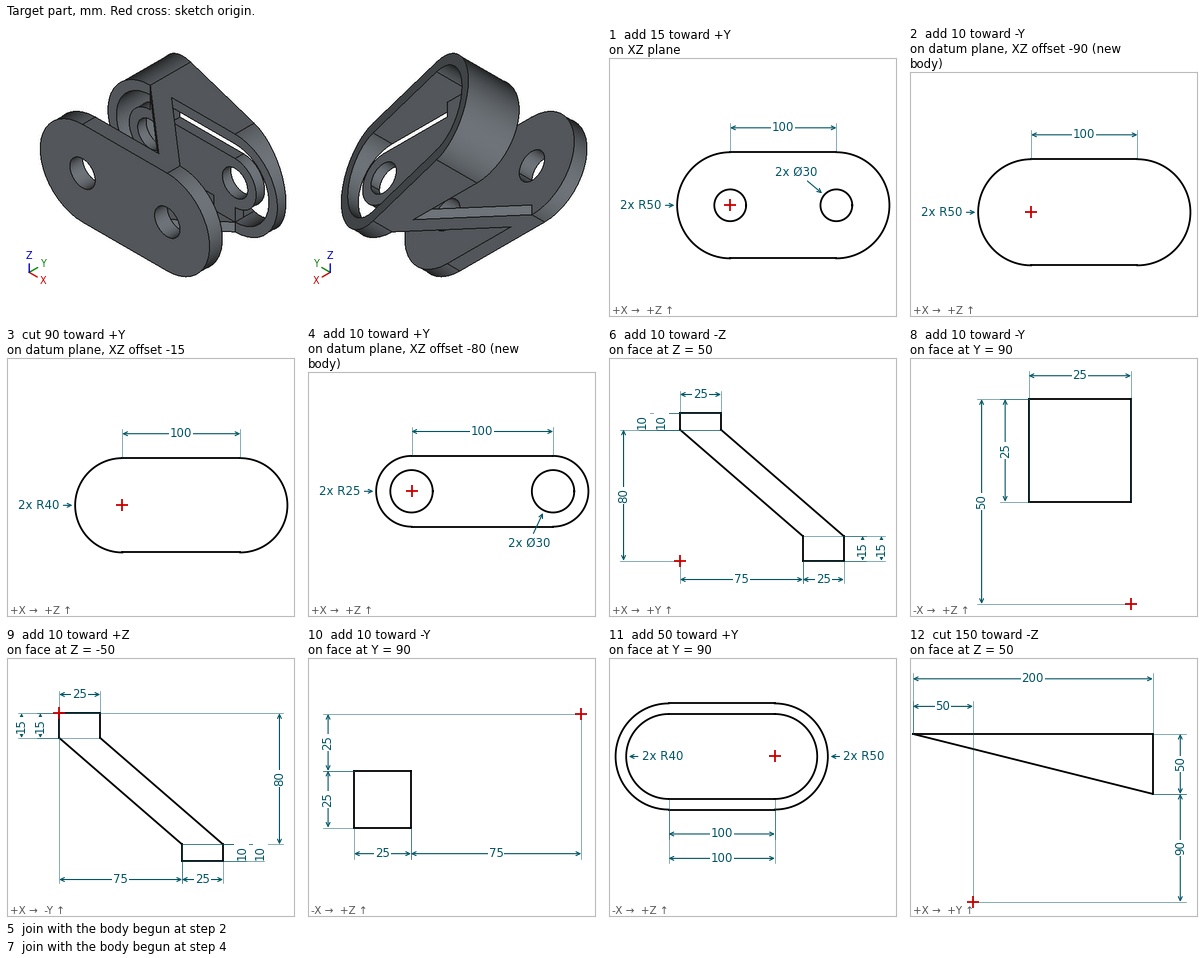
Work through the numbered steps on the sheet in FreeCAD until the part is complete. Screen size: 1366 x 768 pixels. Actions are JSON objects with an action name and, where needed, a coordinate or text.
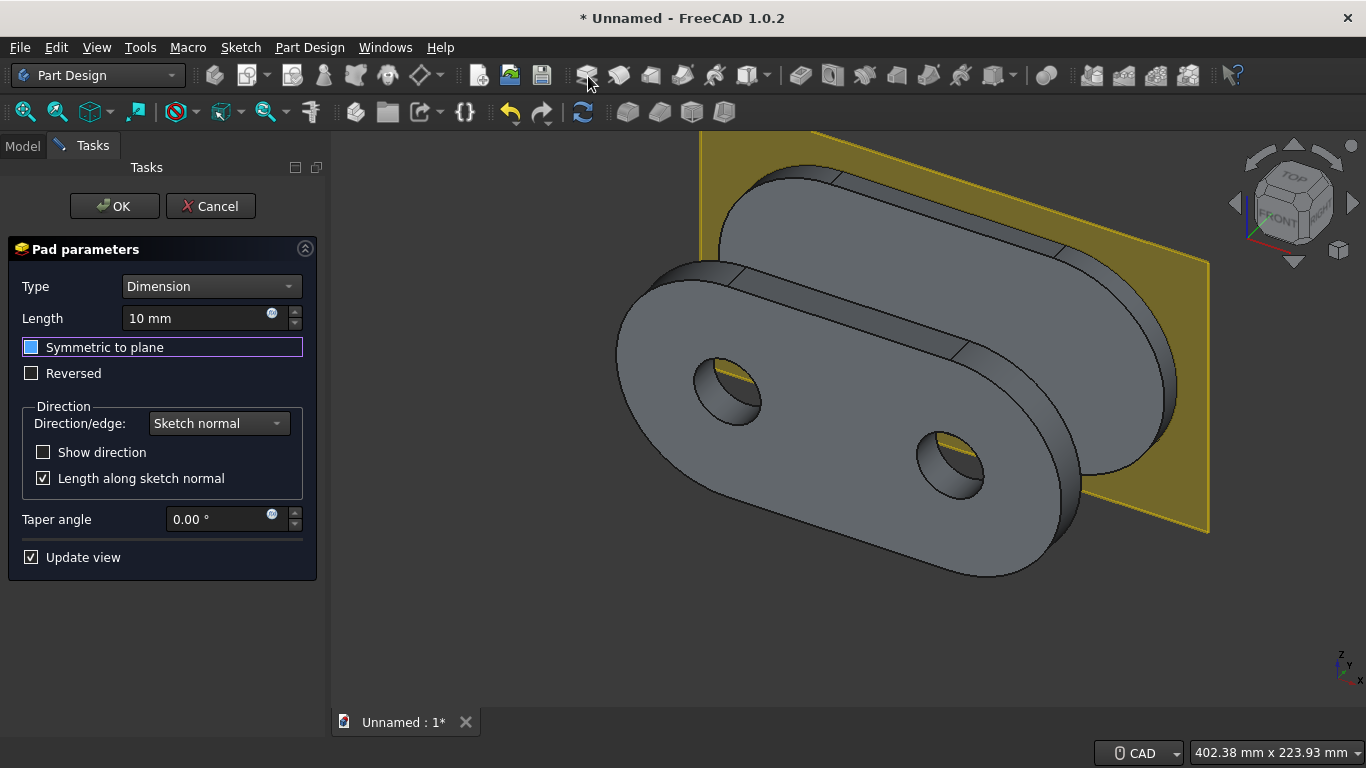
{"action": "left_click", "coordinate": [115, 206]}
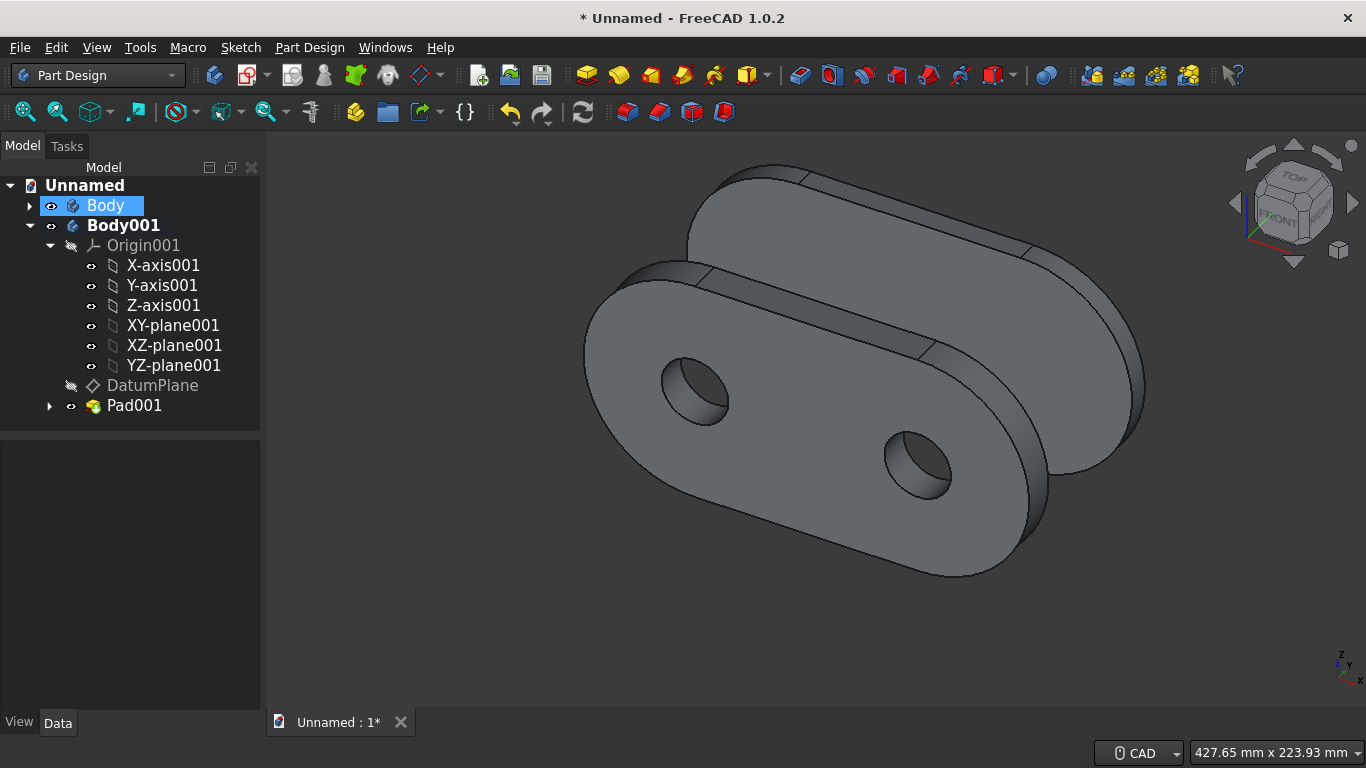
{"action": "left_click", "coordinate": [136, 346]}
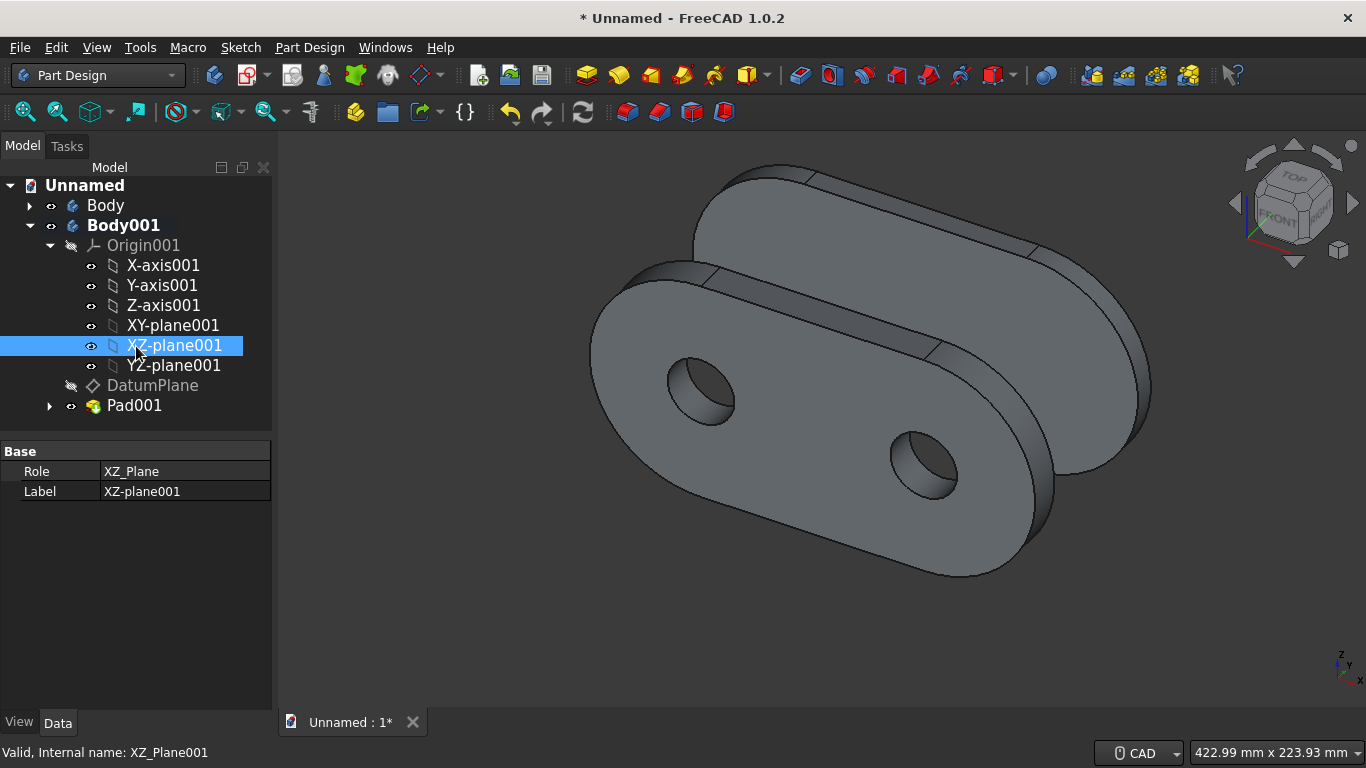
{"action": "left_click", "coordinate": [420, 76]}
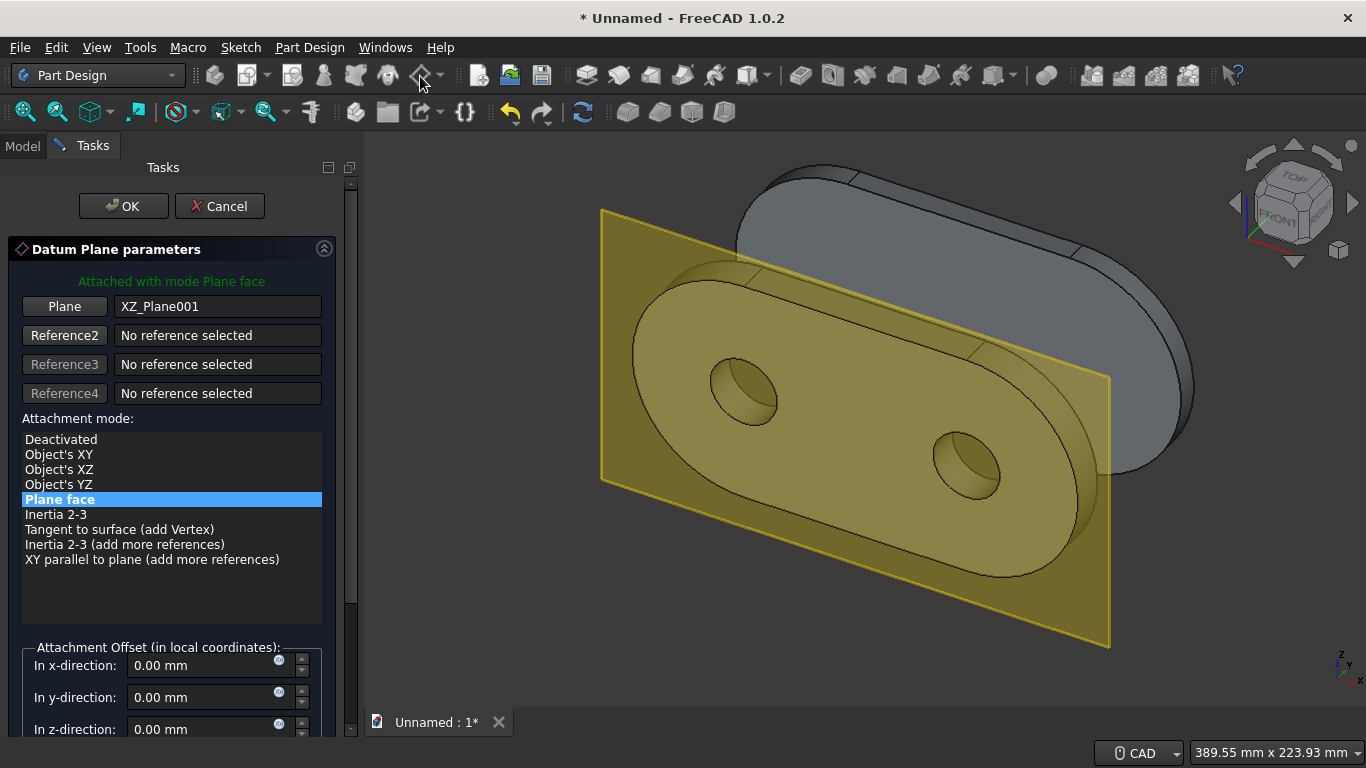
{"action": "scroll", "coordinate": [351, 456], "scroll_direction": "down", "scroll_amount": 2}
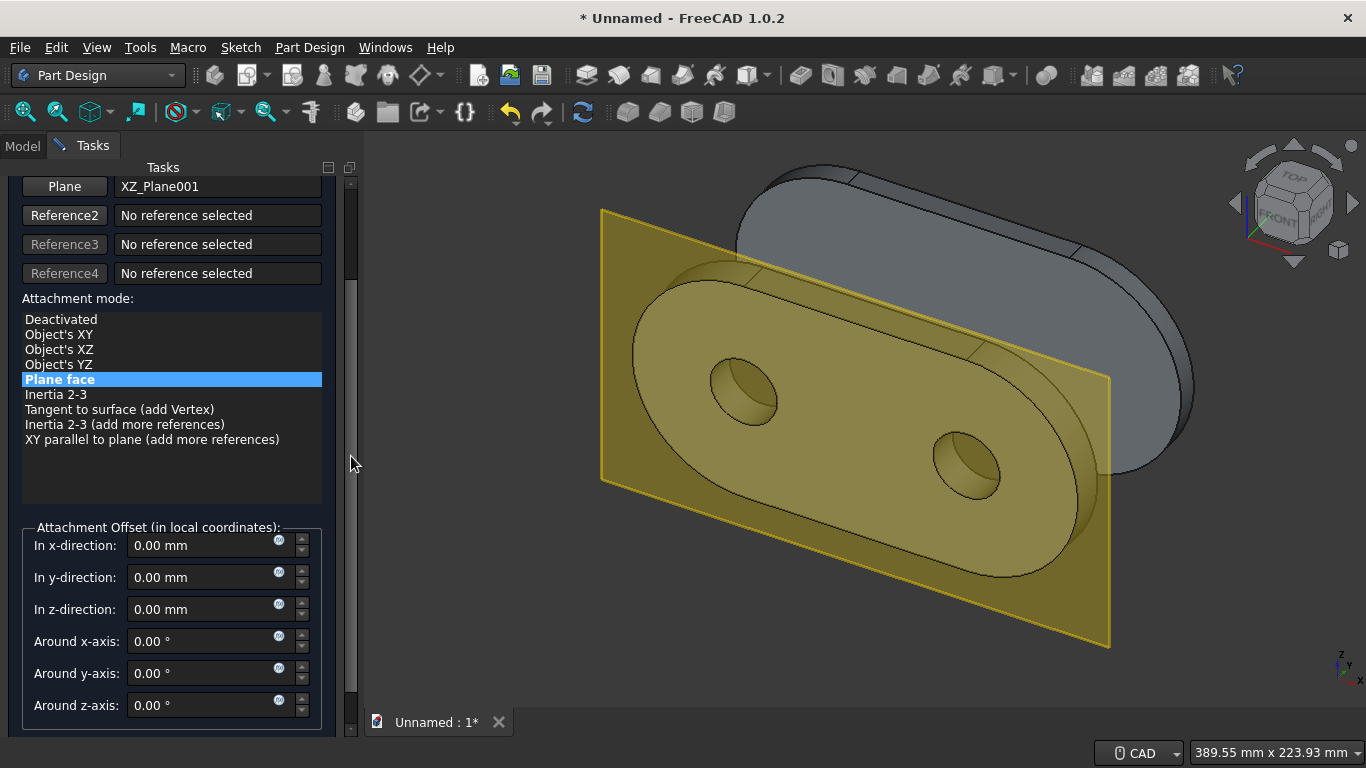
{"action": "triple_click", "coordinate": [210, 609]}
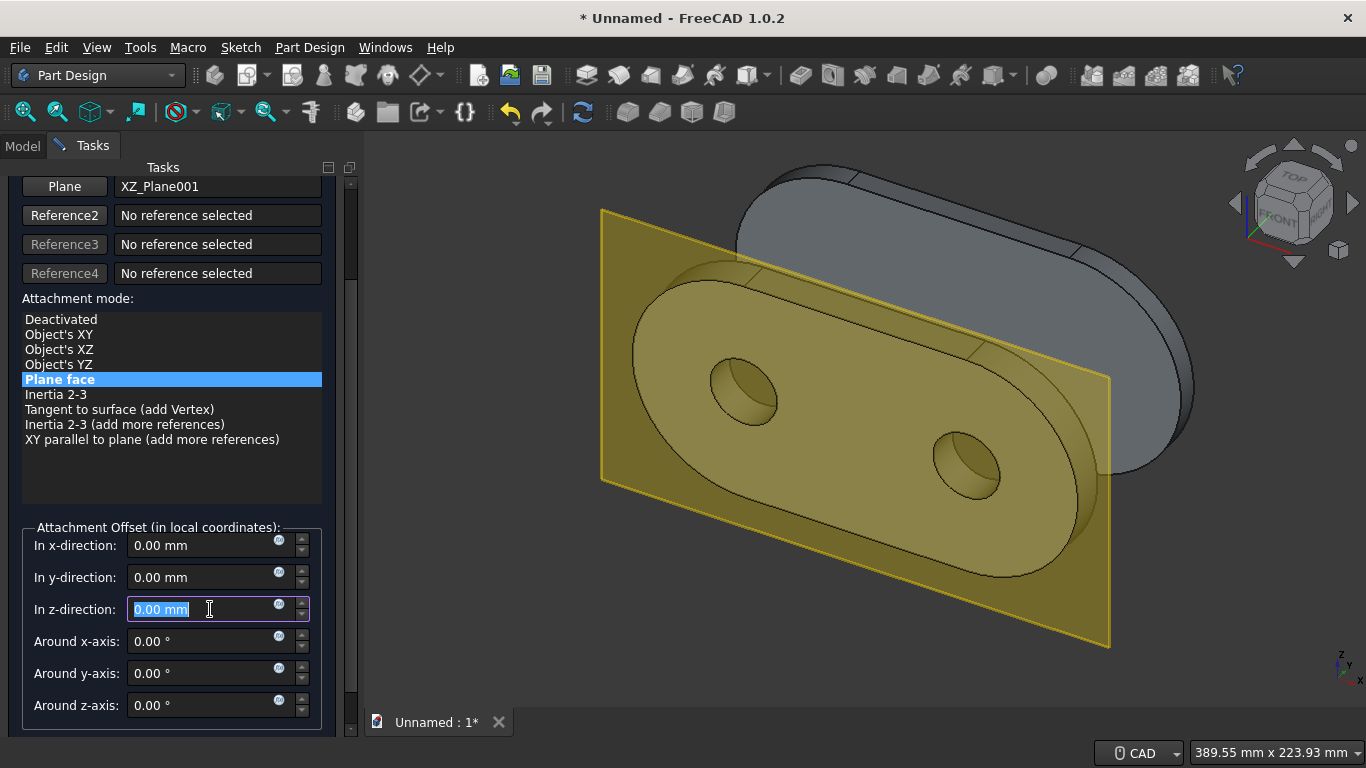
{"action": "type", "text": "-15"}
{"action": "key", "text": "Tab"}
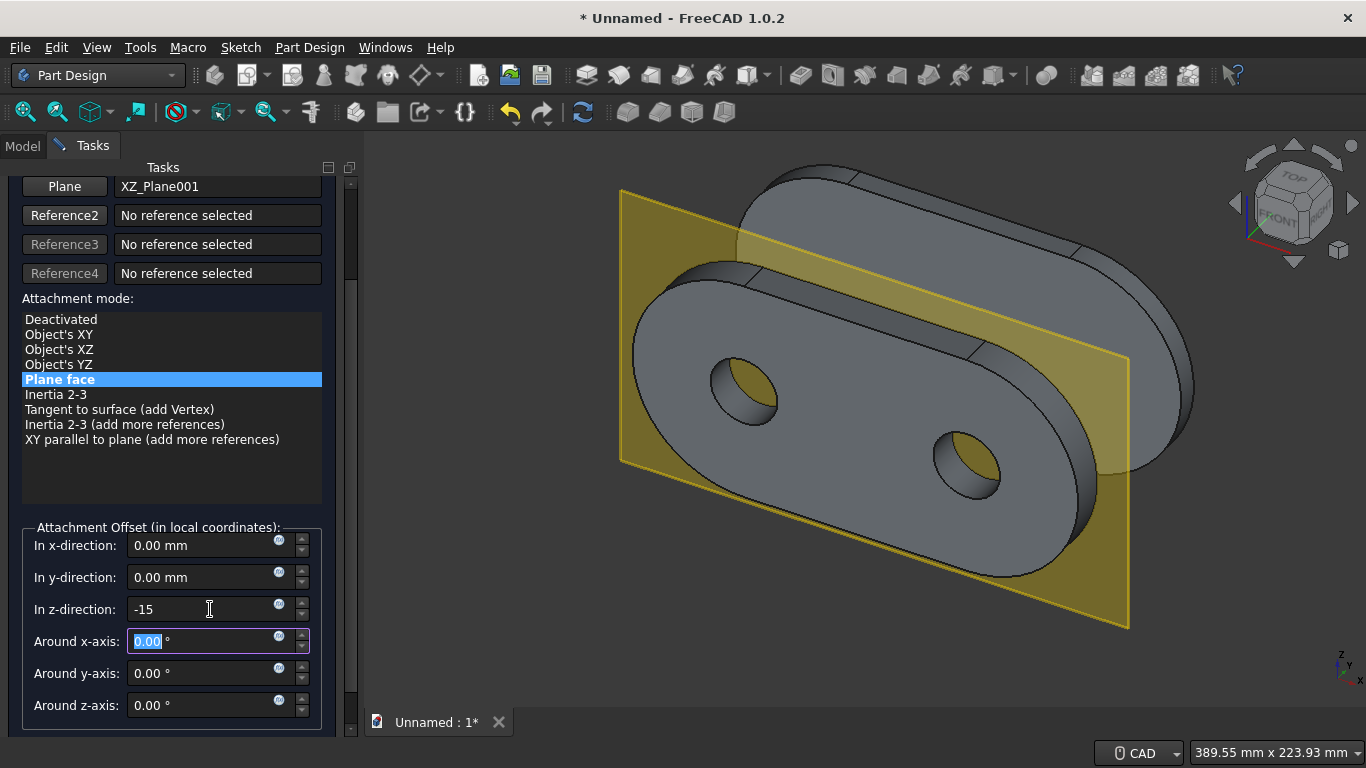
{"action": "scroll", "coordinate": [351, 456], "scroll_direction": "up", "scroll_amount": 3}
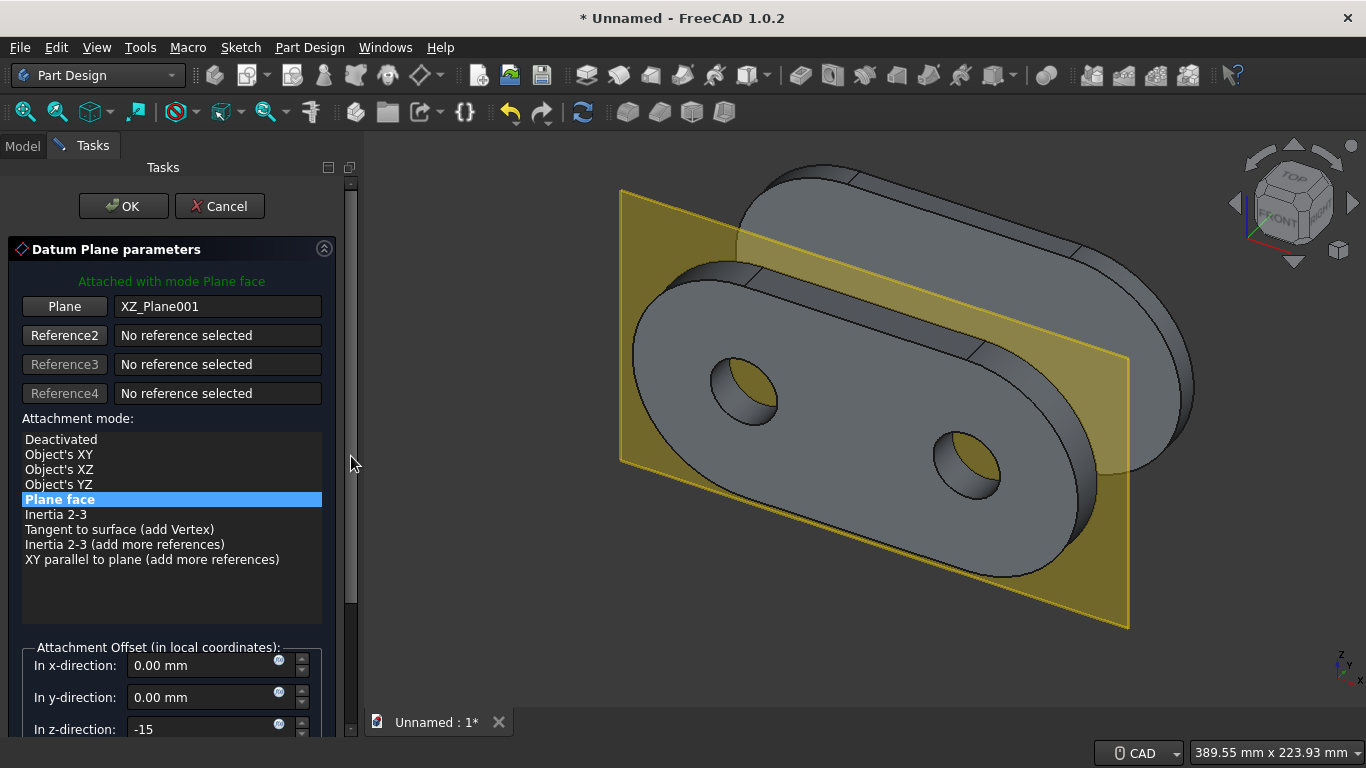
{"action": "left_click", "coordinate": [124, 206]}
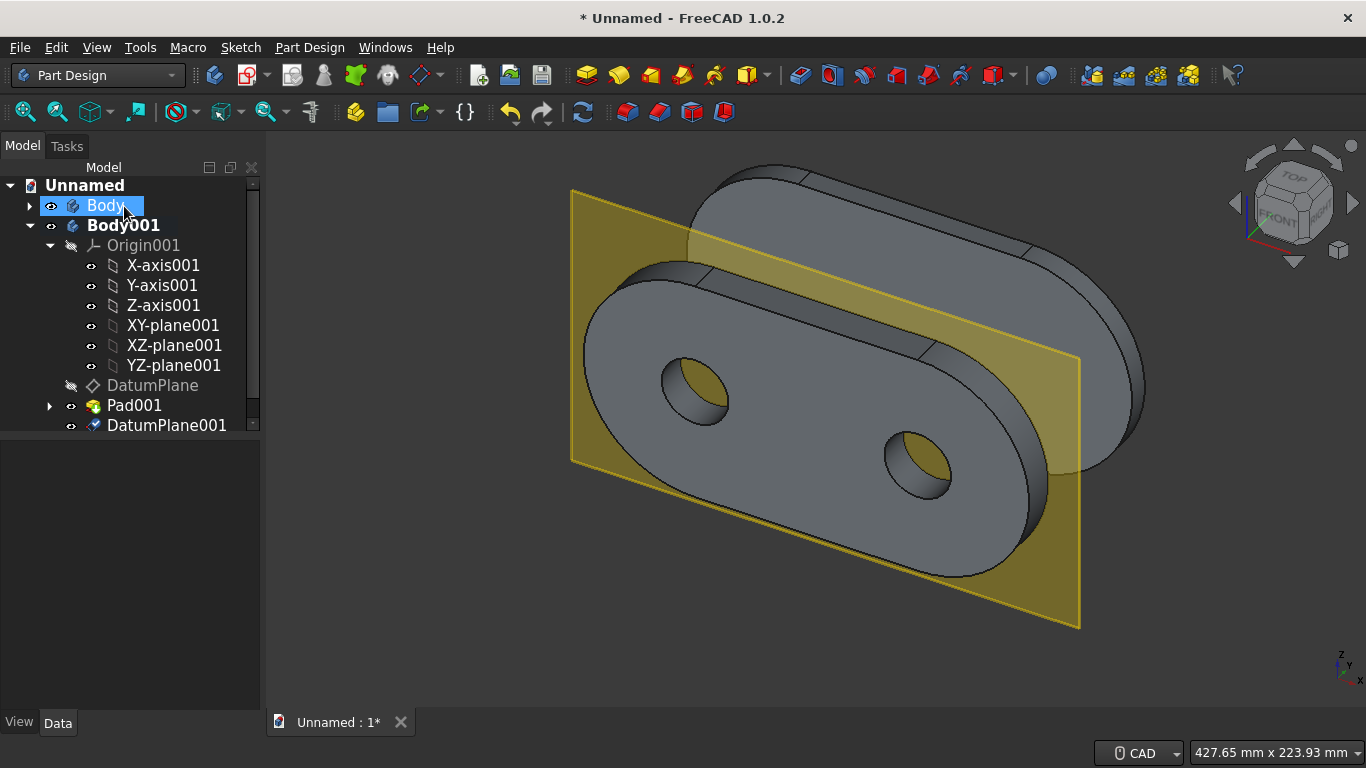
{"action": "left_click", "coordinate": [116, 426]}